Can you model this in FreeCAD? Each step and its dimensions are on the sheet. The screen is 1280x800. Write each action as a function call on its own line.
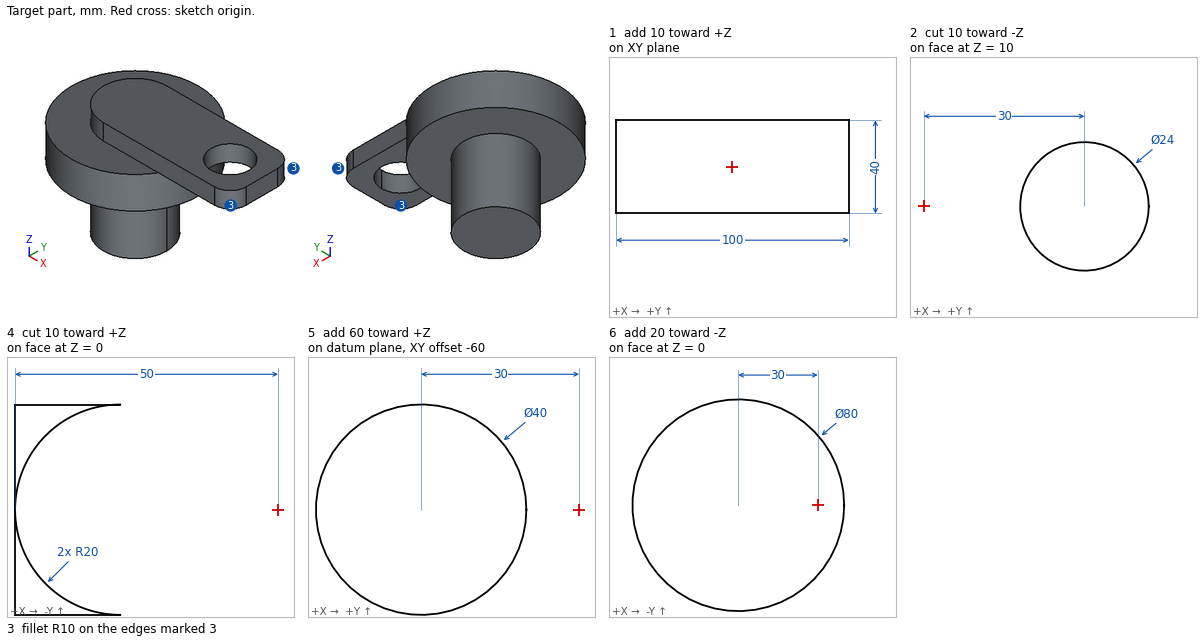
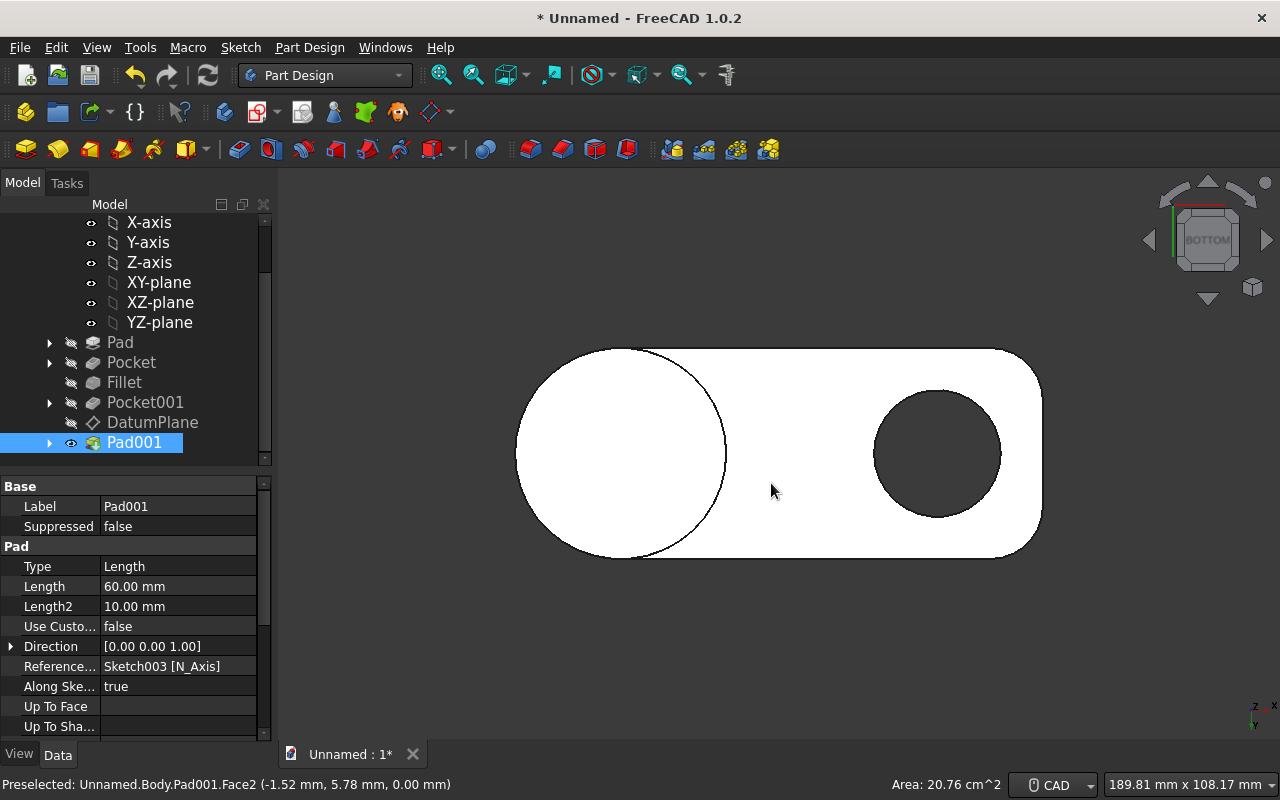
click(258, 112)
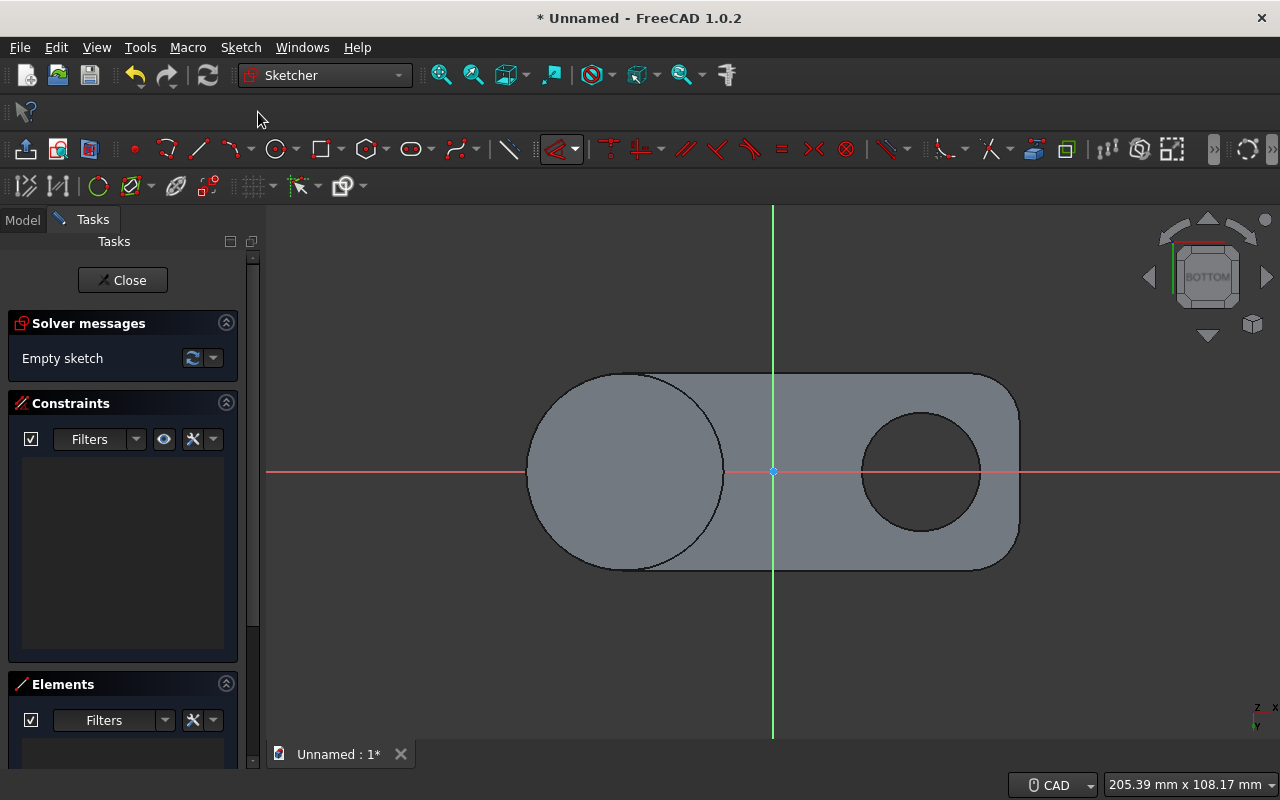
key(g)
key(c)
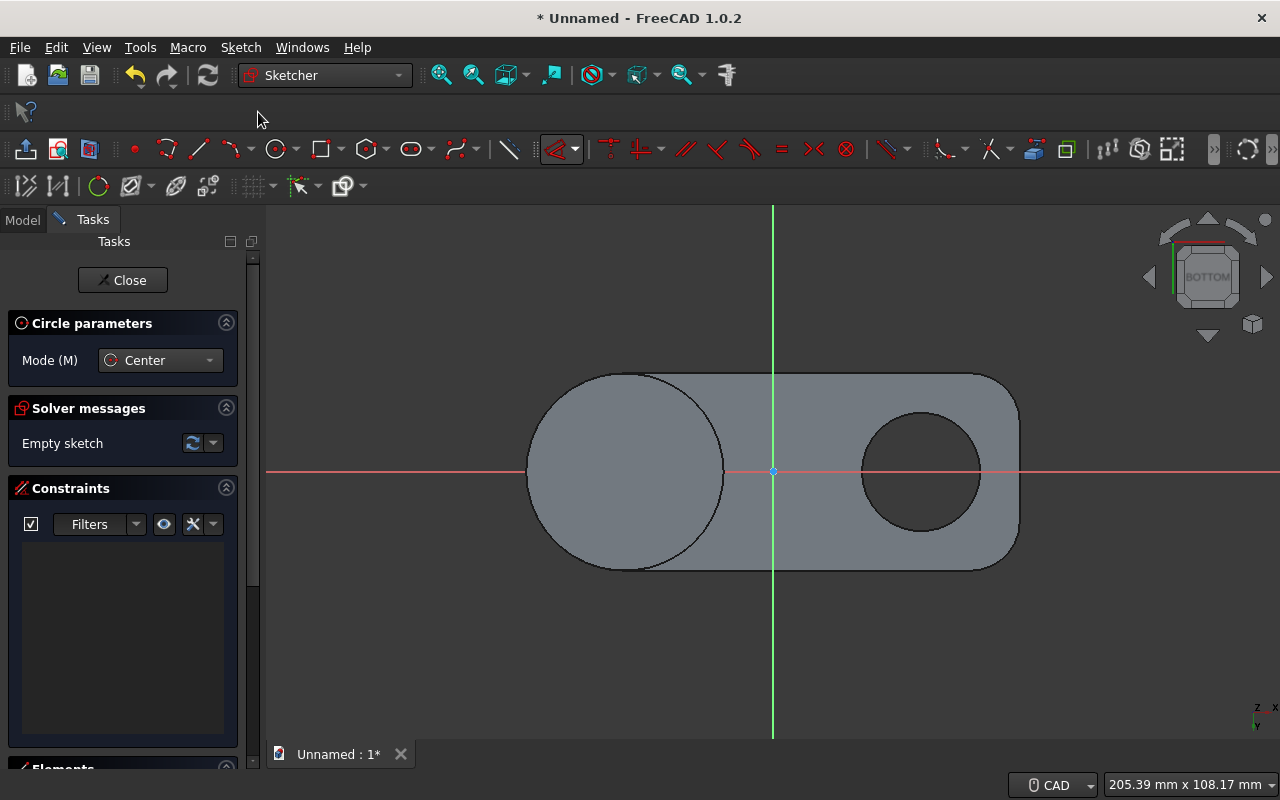
click(625, 472)
move(485, 332)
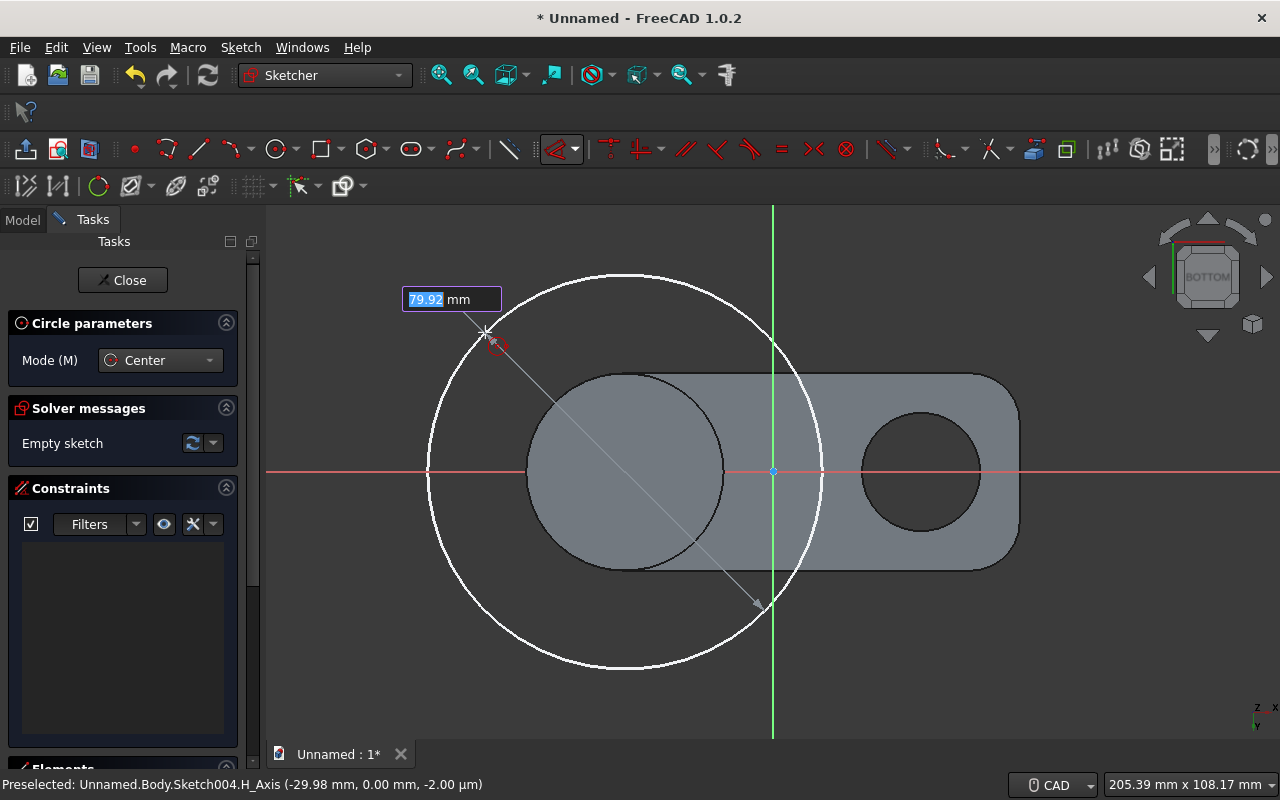
text(80)
key(Return)
key(Escape)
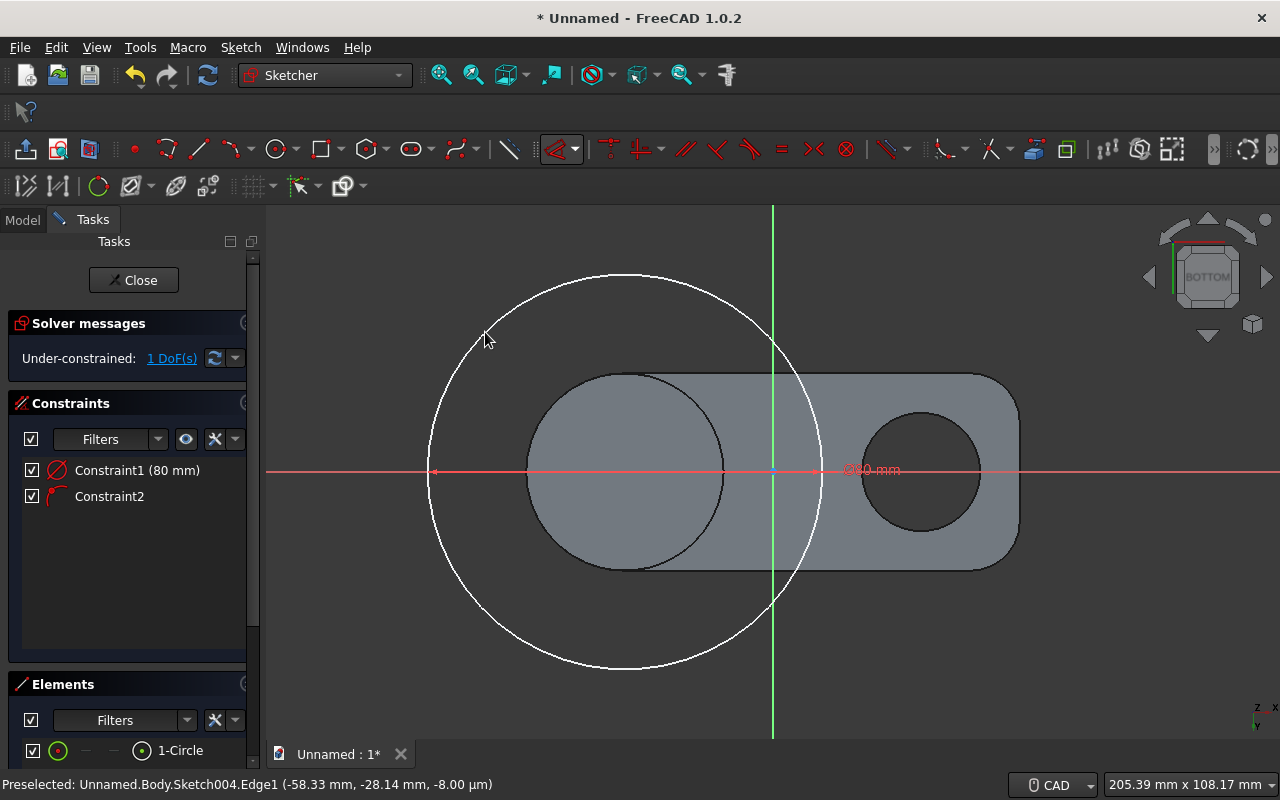
click(625, 472)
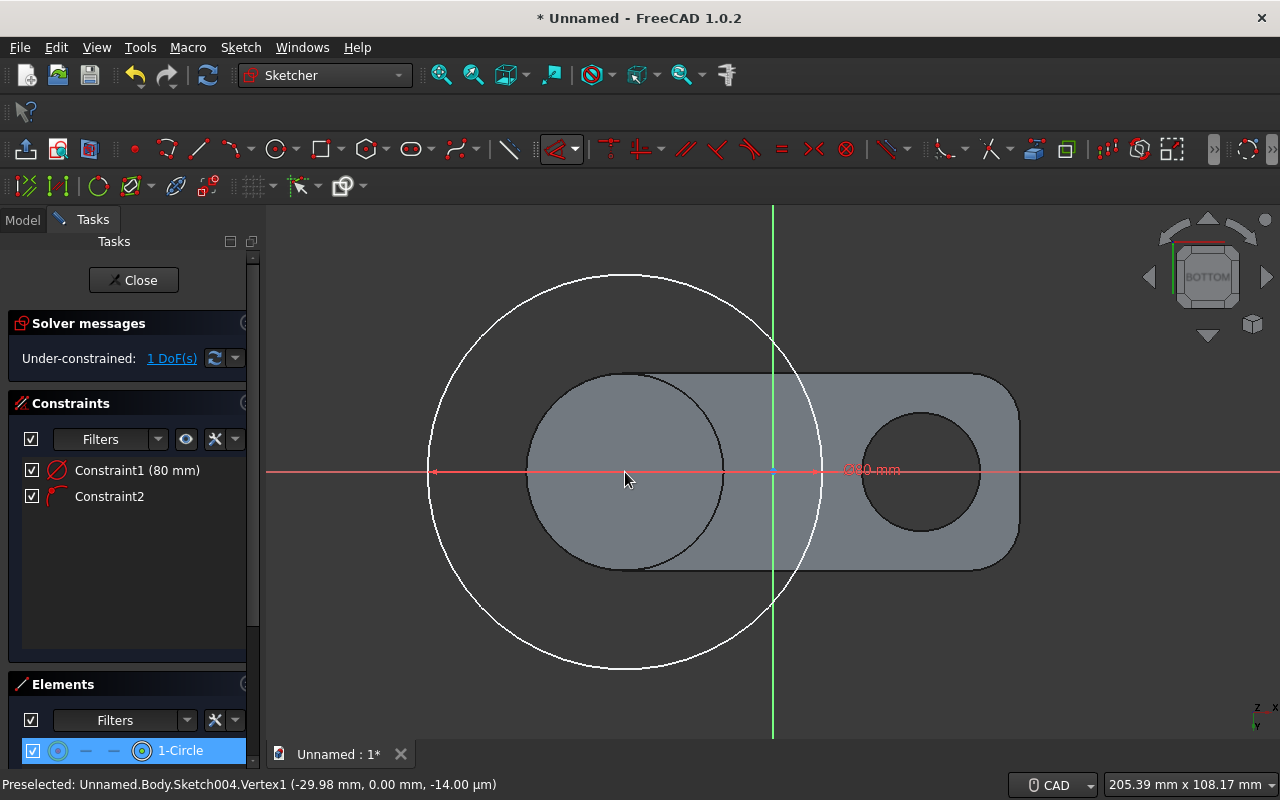
key(l)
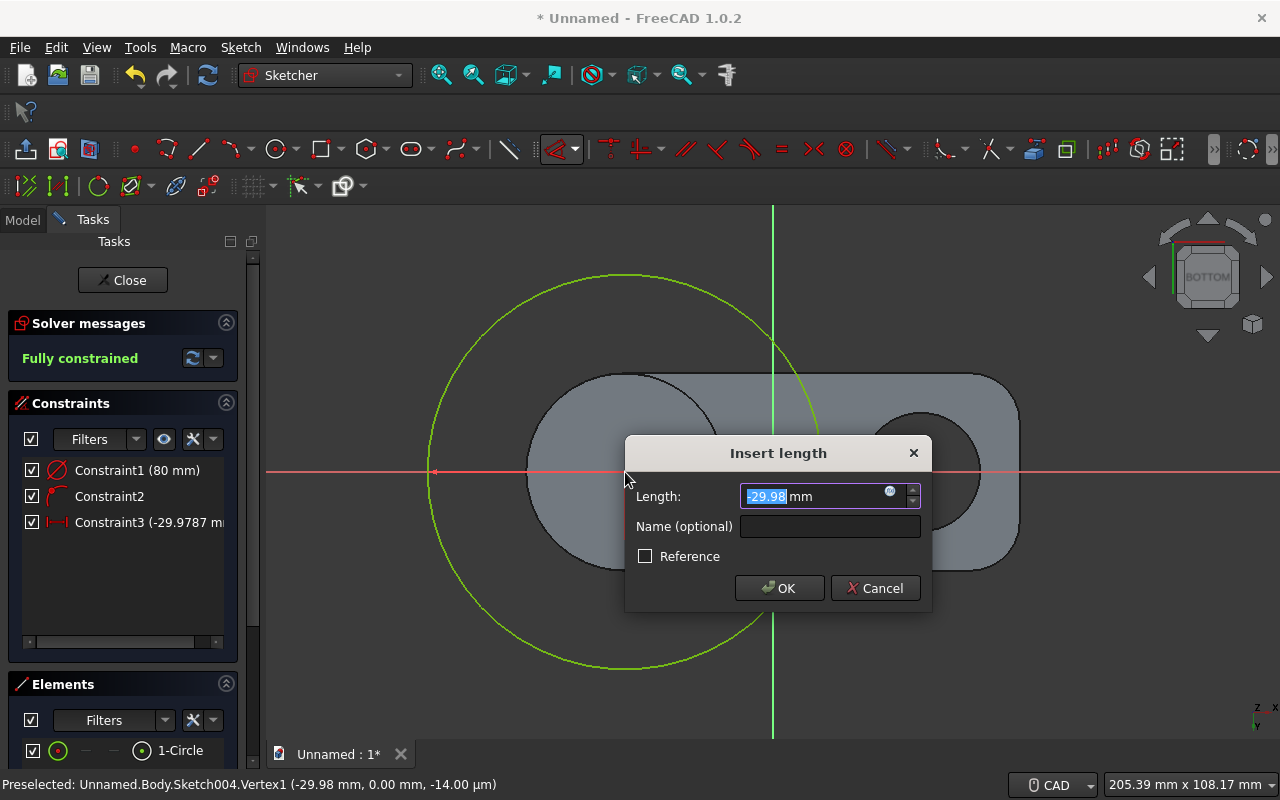
text(-30)
key(Return)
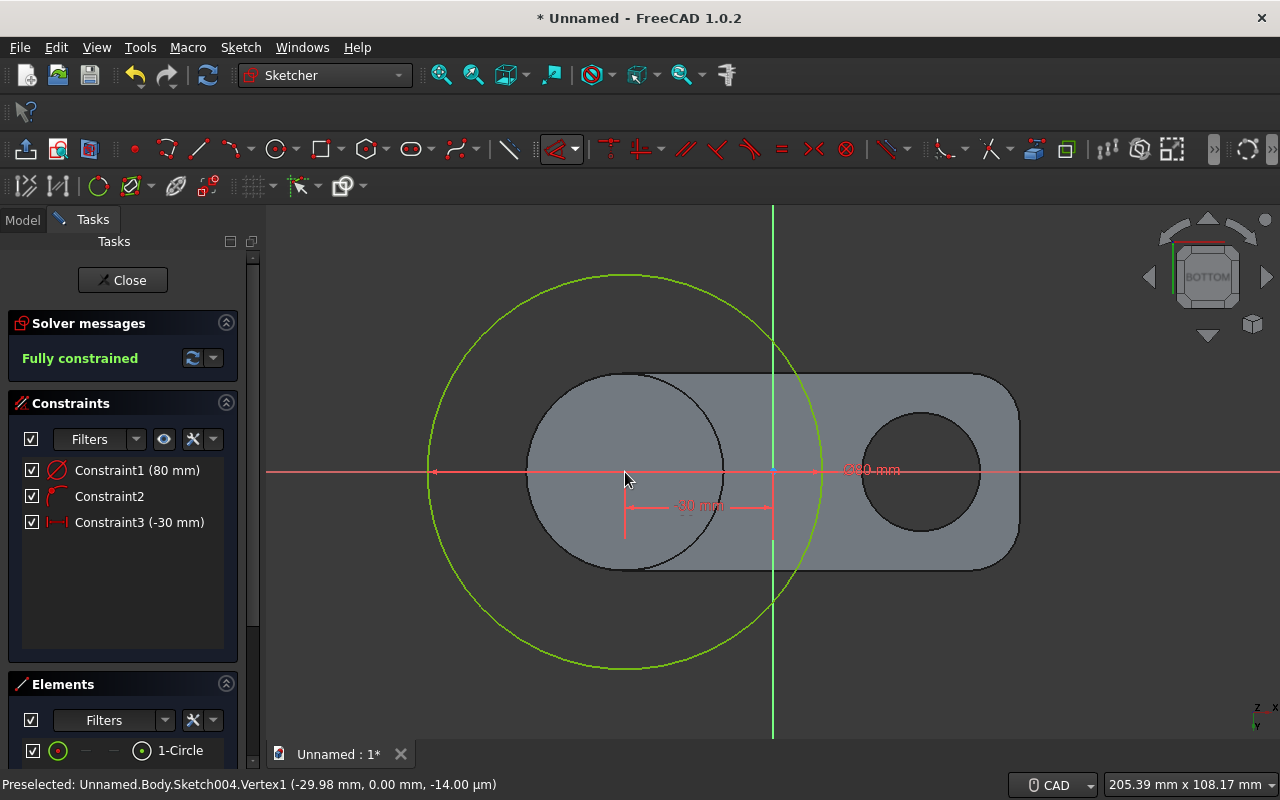
click(123, 280)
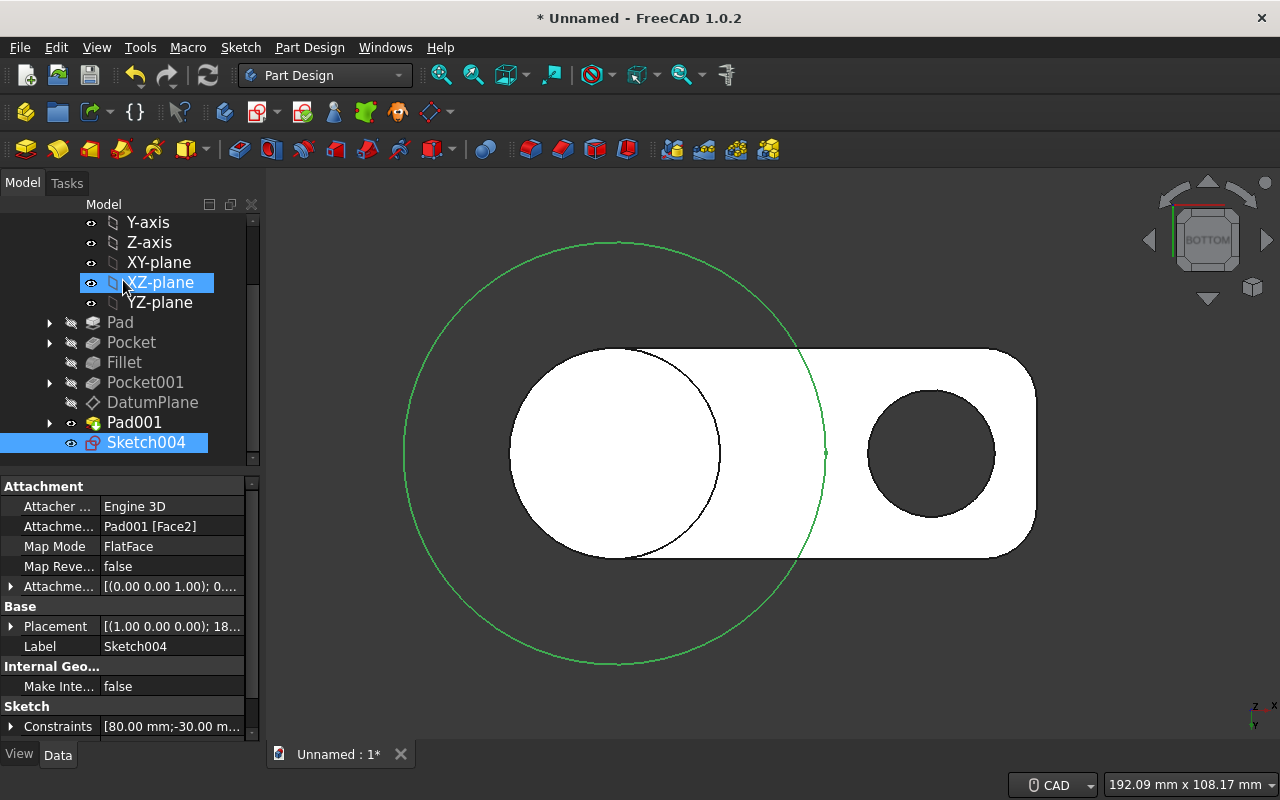
click(26, 150)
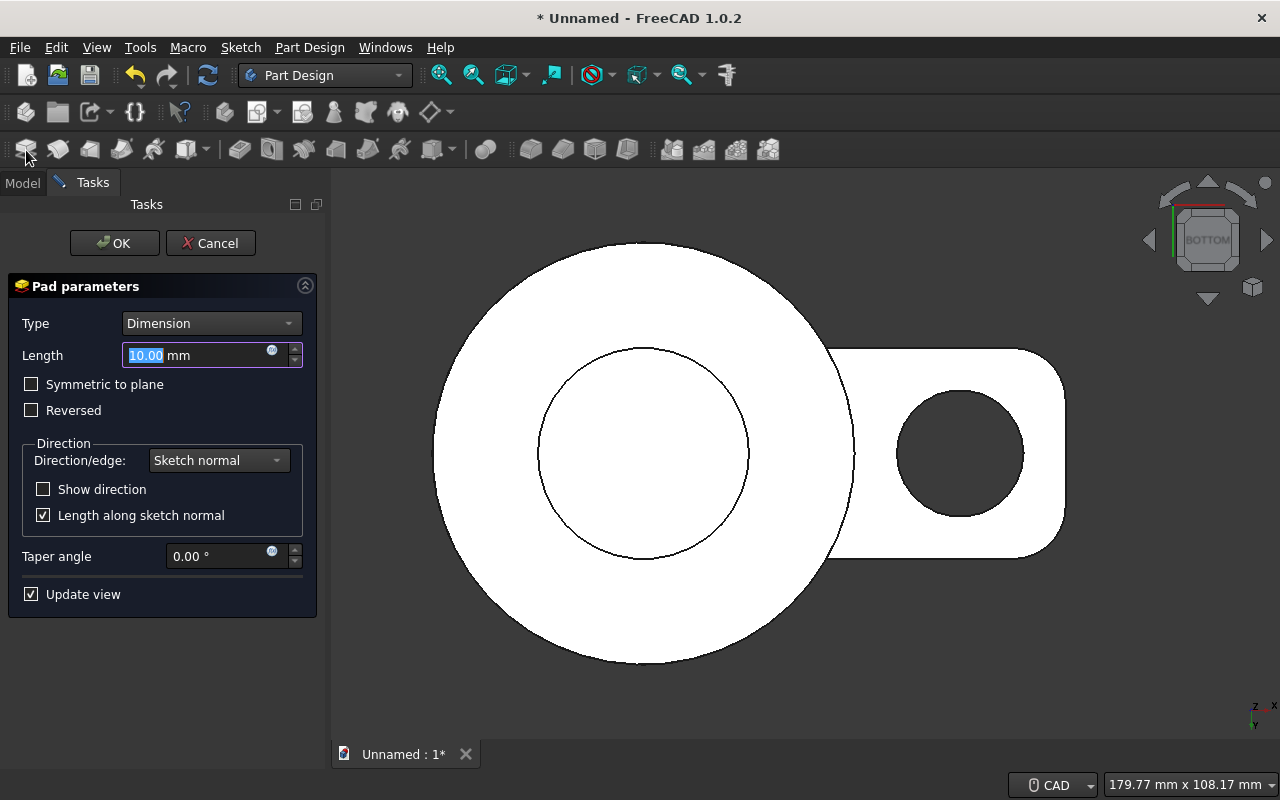
text(20)
key(Tab)